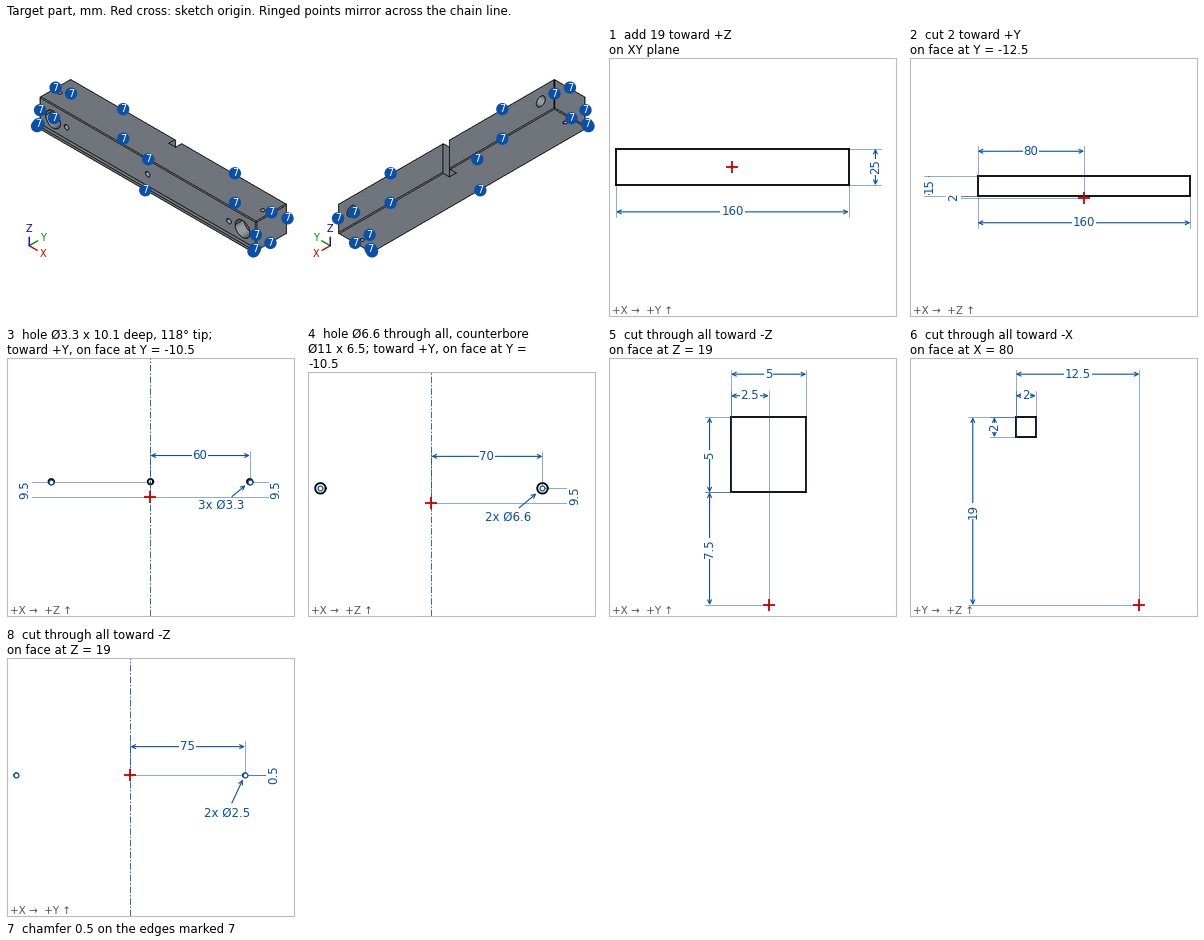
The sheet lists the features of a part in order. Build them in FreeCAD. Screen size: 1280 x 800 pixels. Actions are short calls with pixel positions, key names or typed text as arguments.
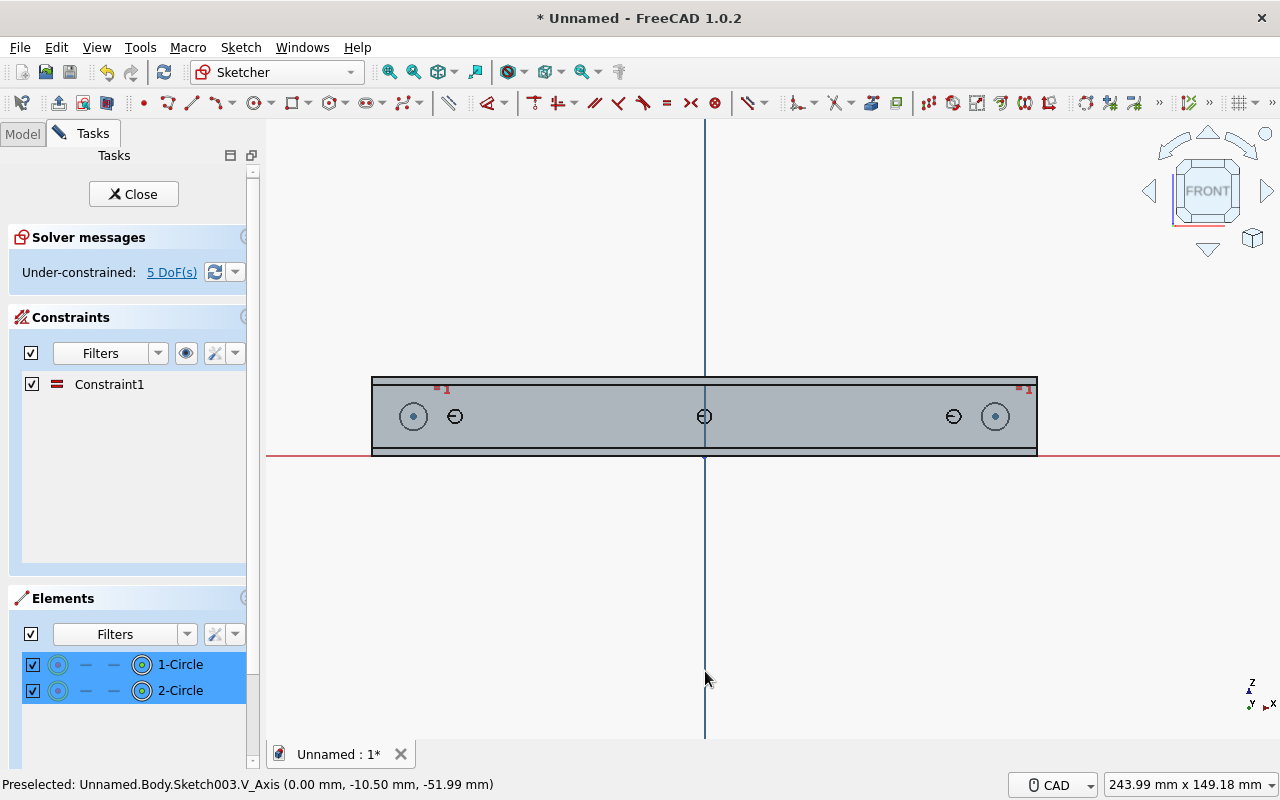
click(692, 104)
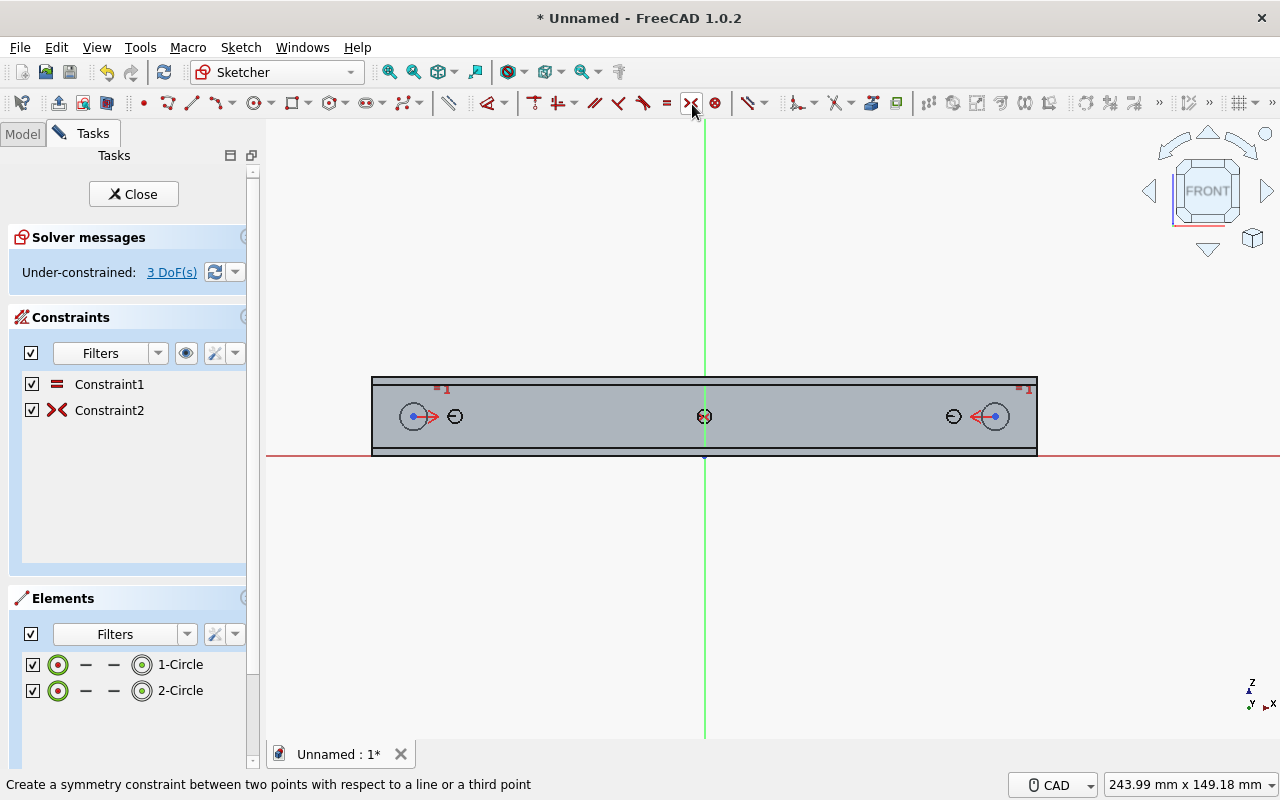
click(488, 104)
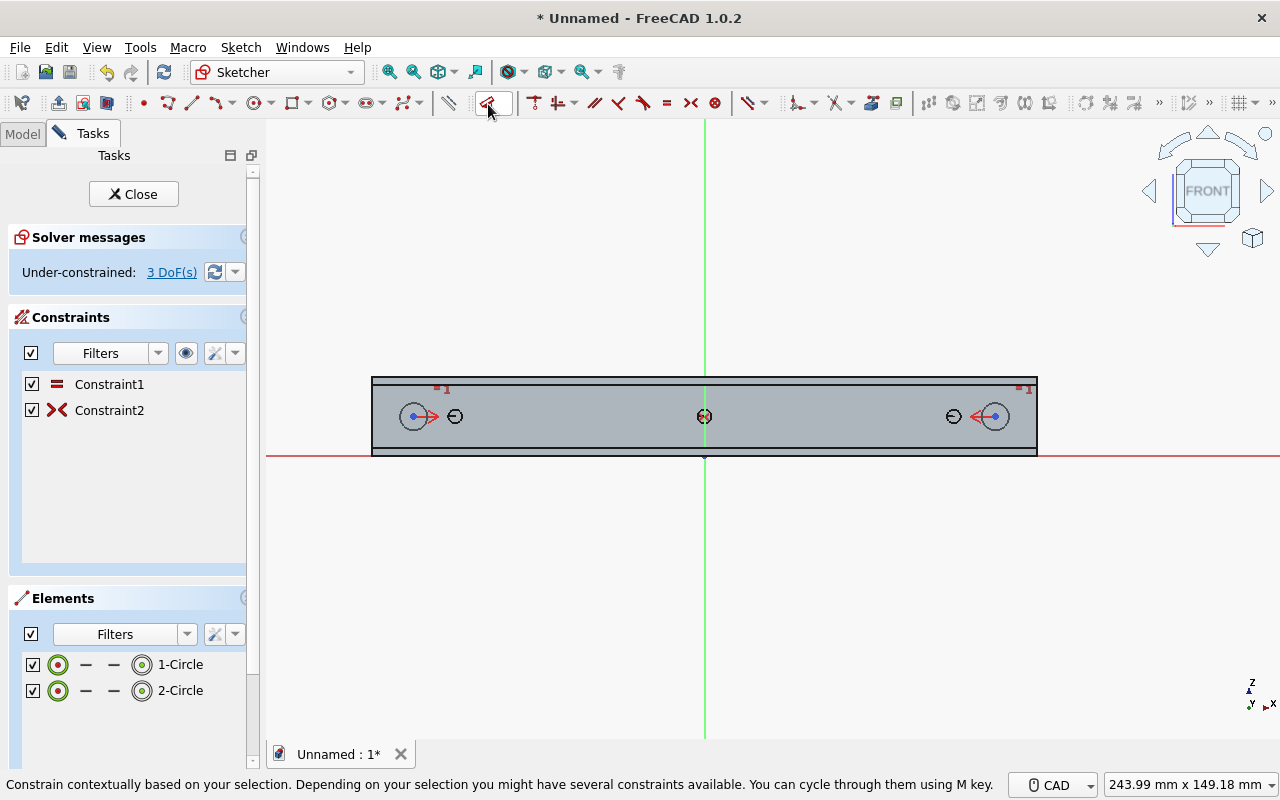
scroll(1005, 407, up, 2)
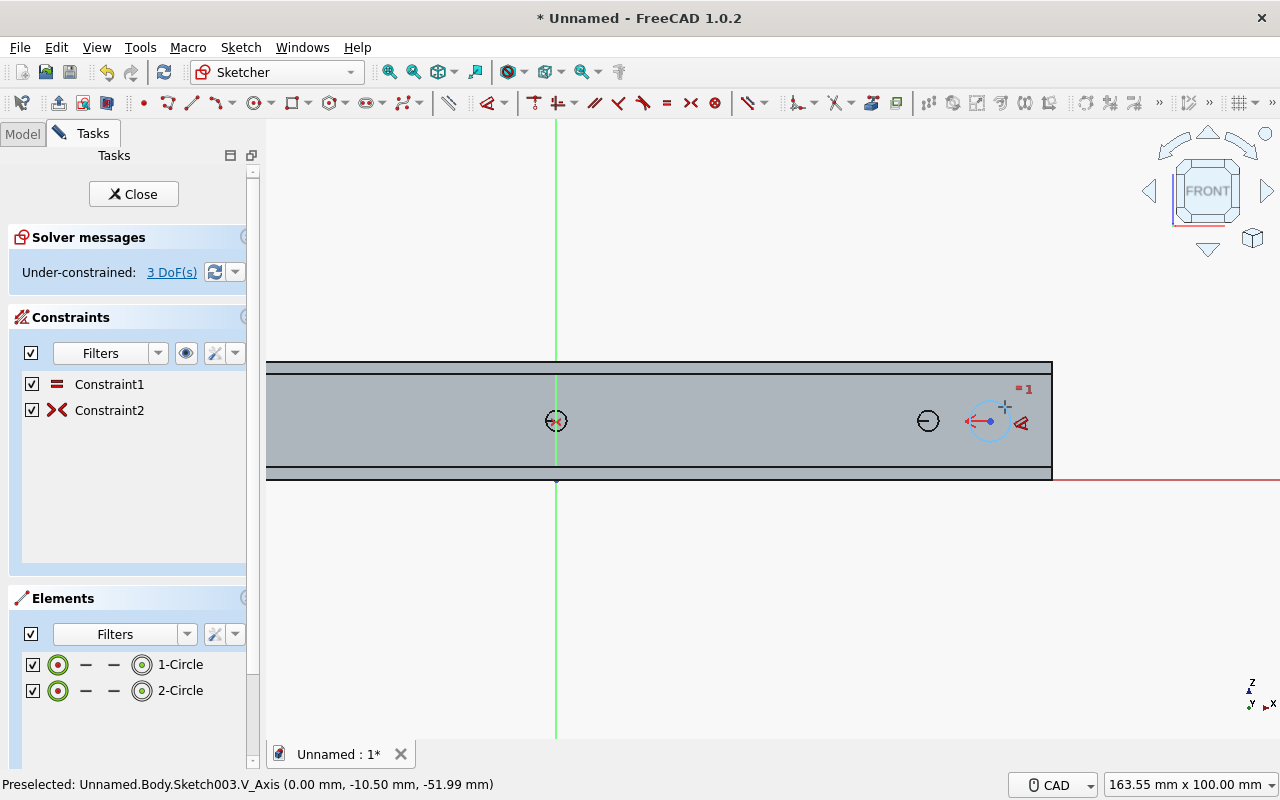
click(1004, 407)
click(1026, 384)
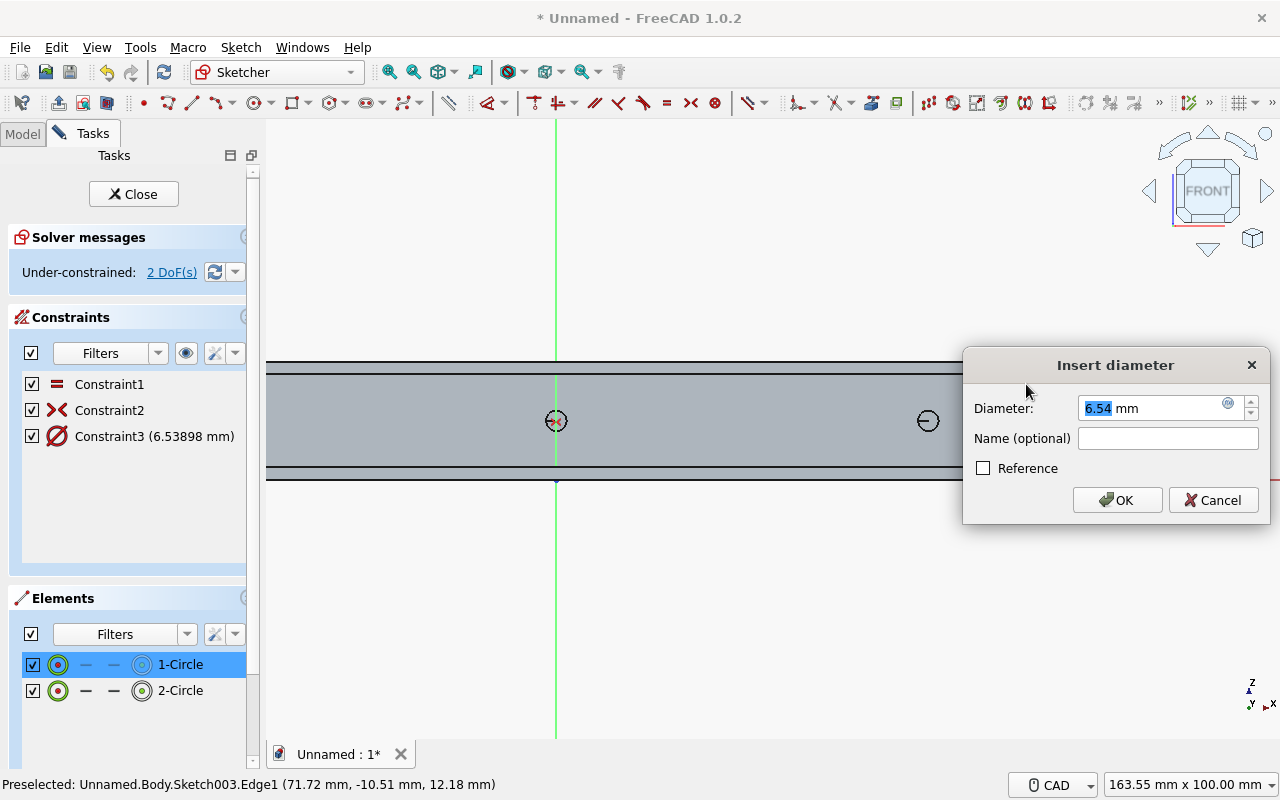
text(6.6)
key(Return)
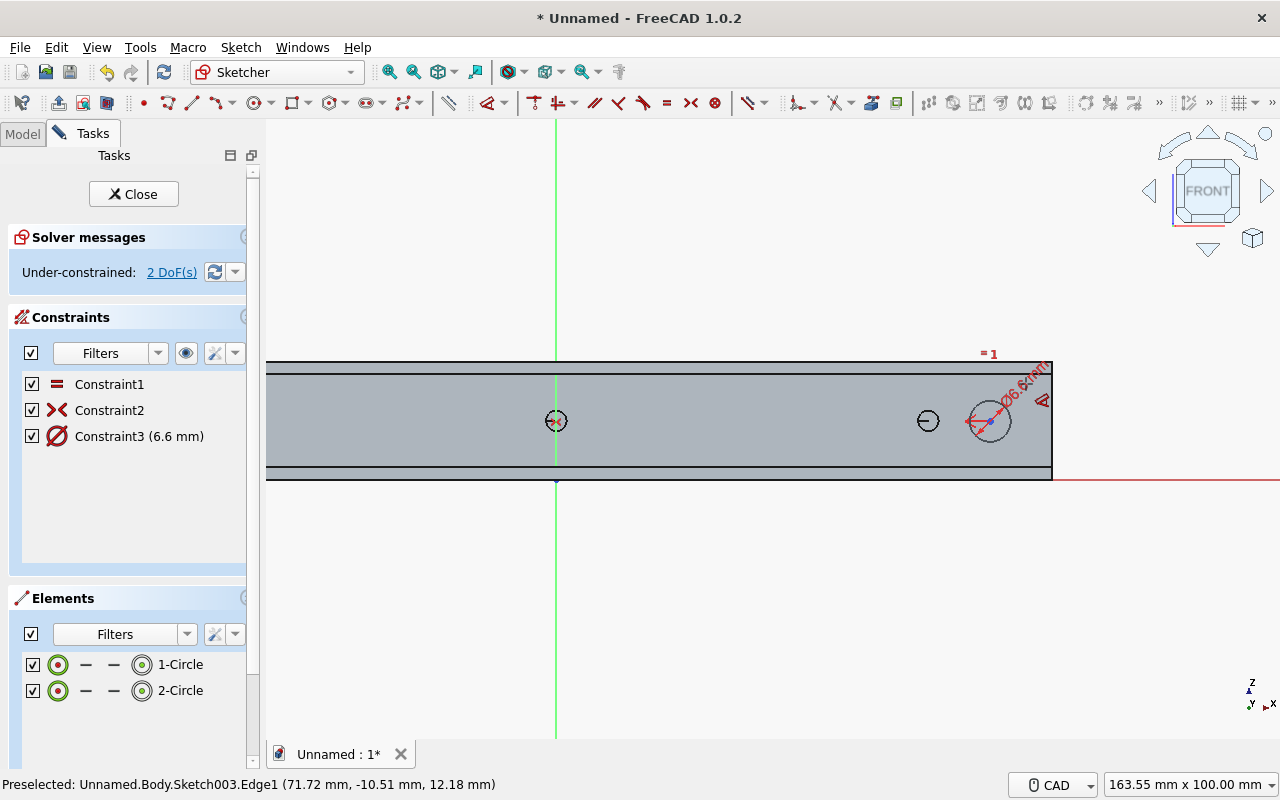
click(990, 421)
click(773, 514)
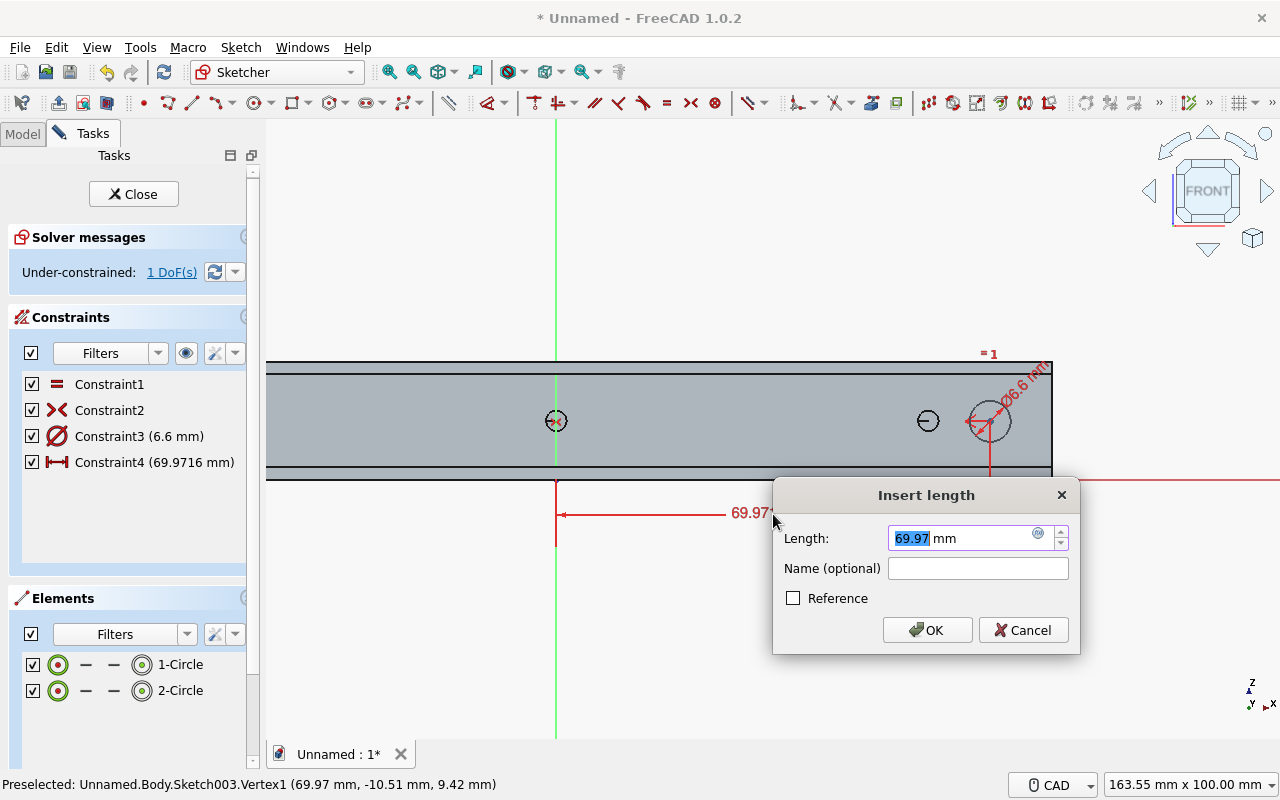
text(70)
key(Return)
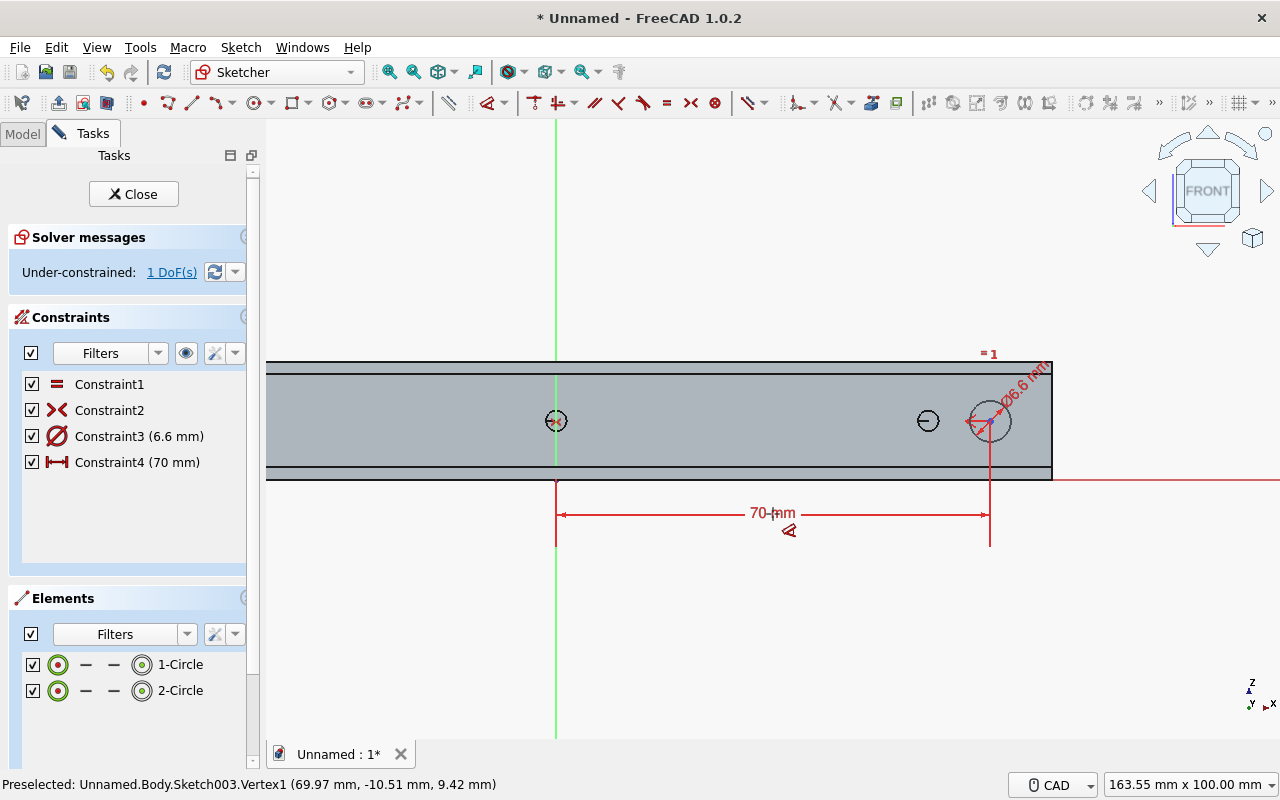
click(990, 421)
click(1024, 451)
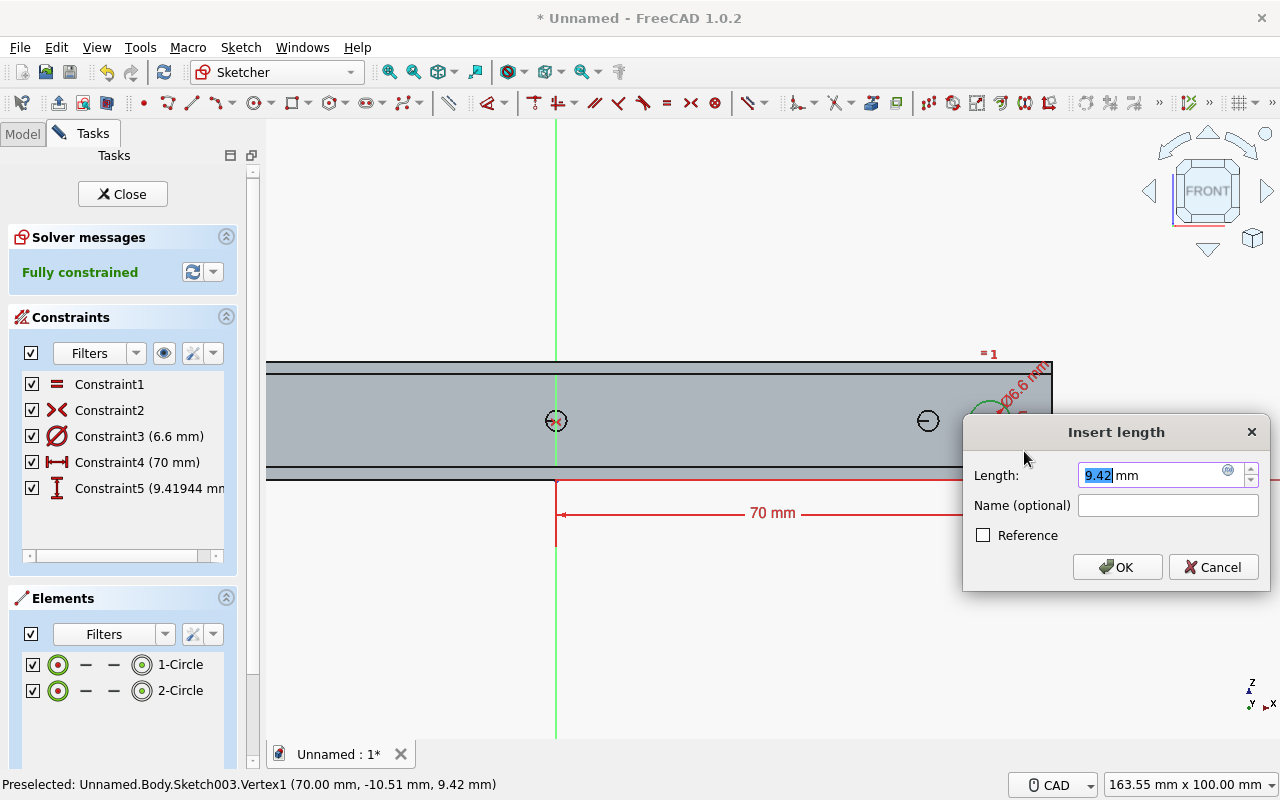
text(9.5)
key(Return)
key(Escape)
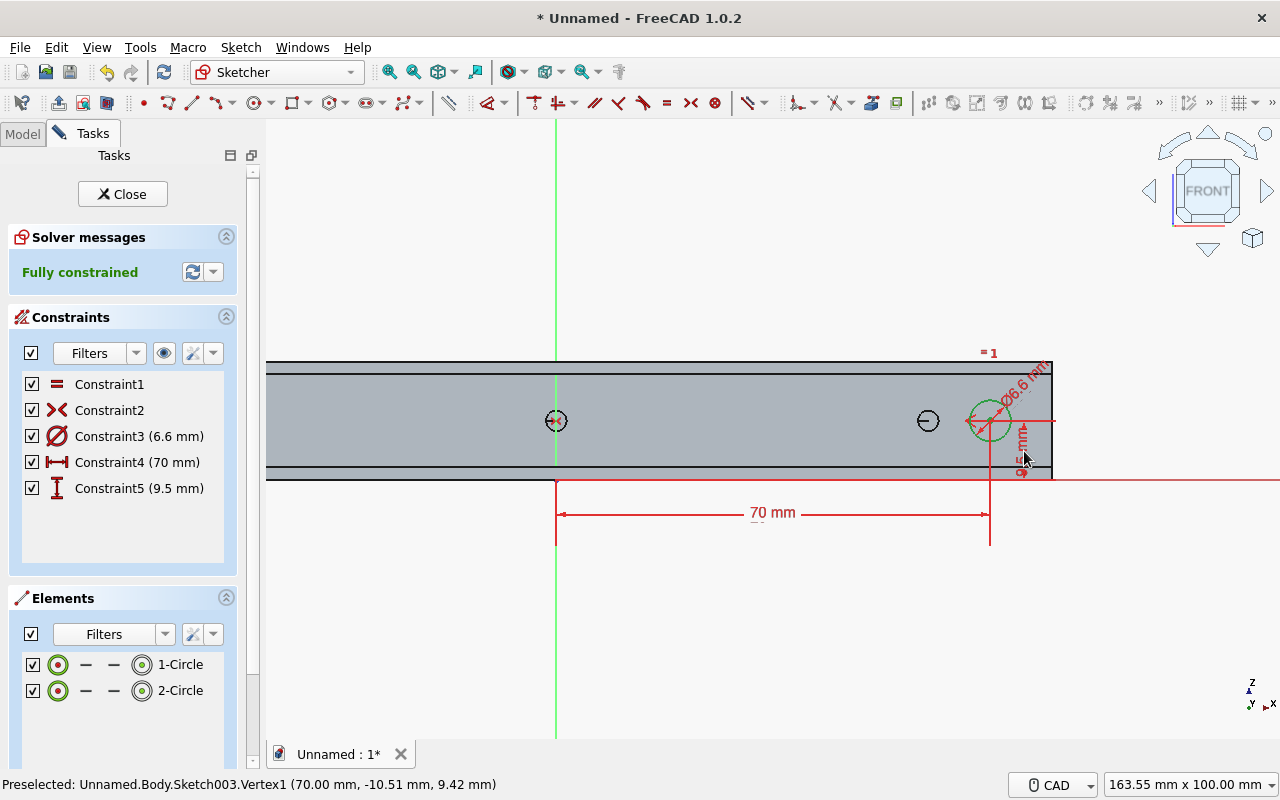
click(123, 194)